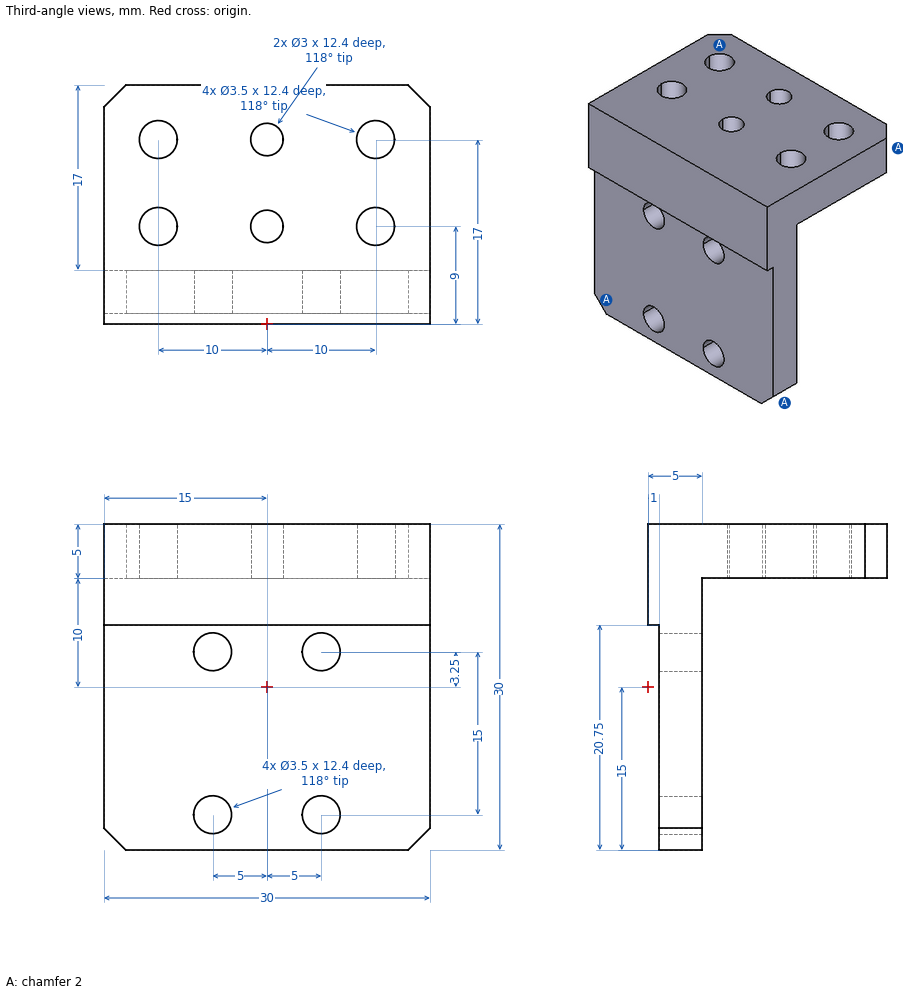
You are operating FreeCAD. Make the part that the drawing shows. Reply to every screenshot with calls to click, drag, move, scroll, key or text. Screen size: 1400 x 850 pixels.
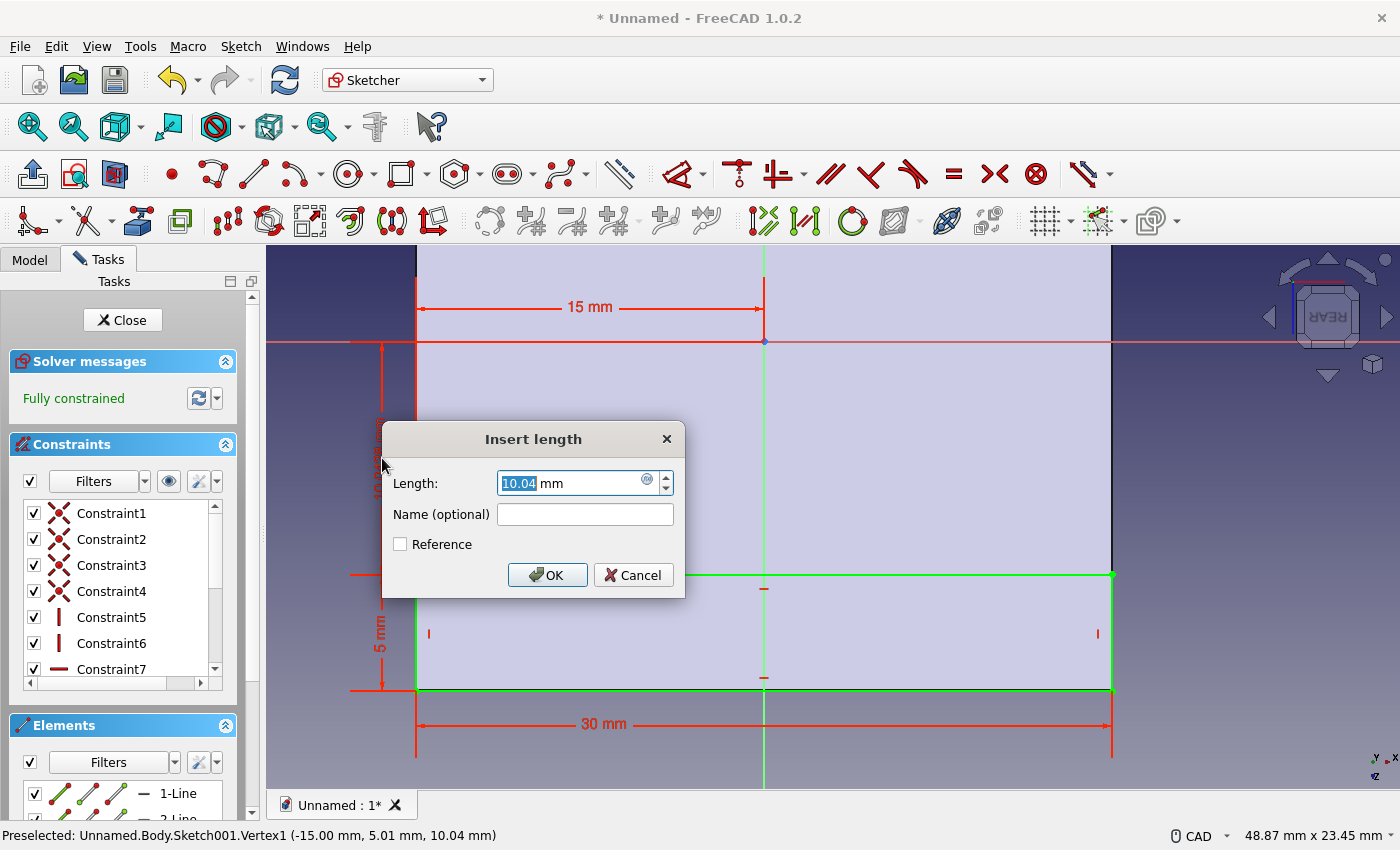
text(10)
key(Return)
key(Escape)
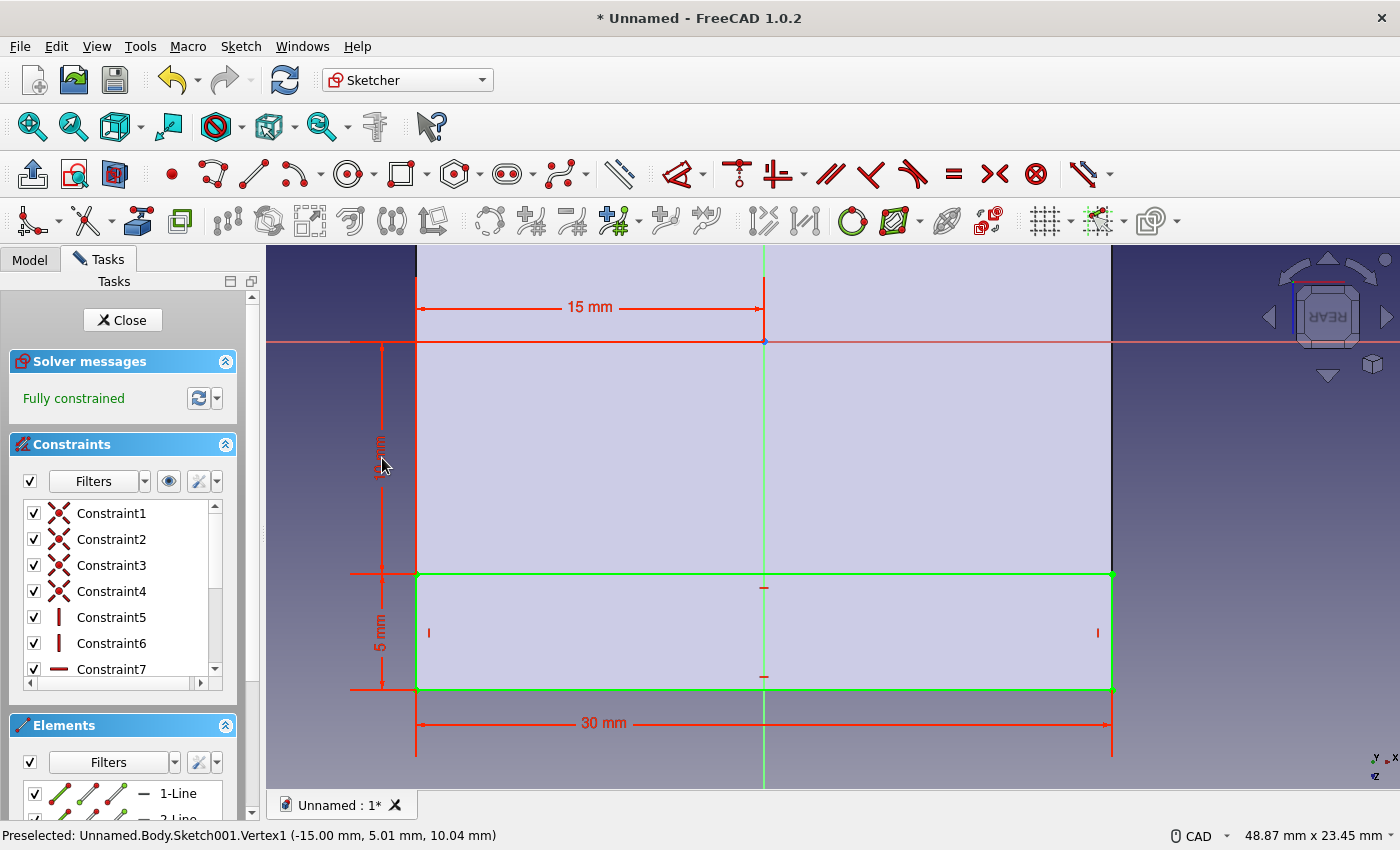
click(123, 320)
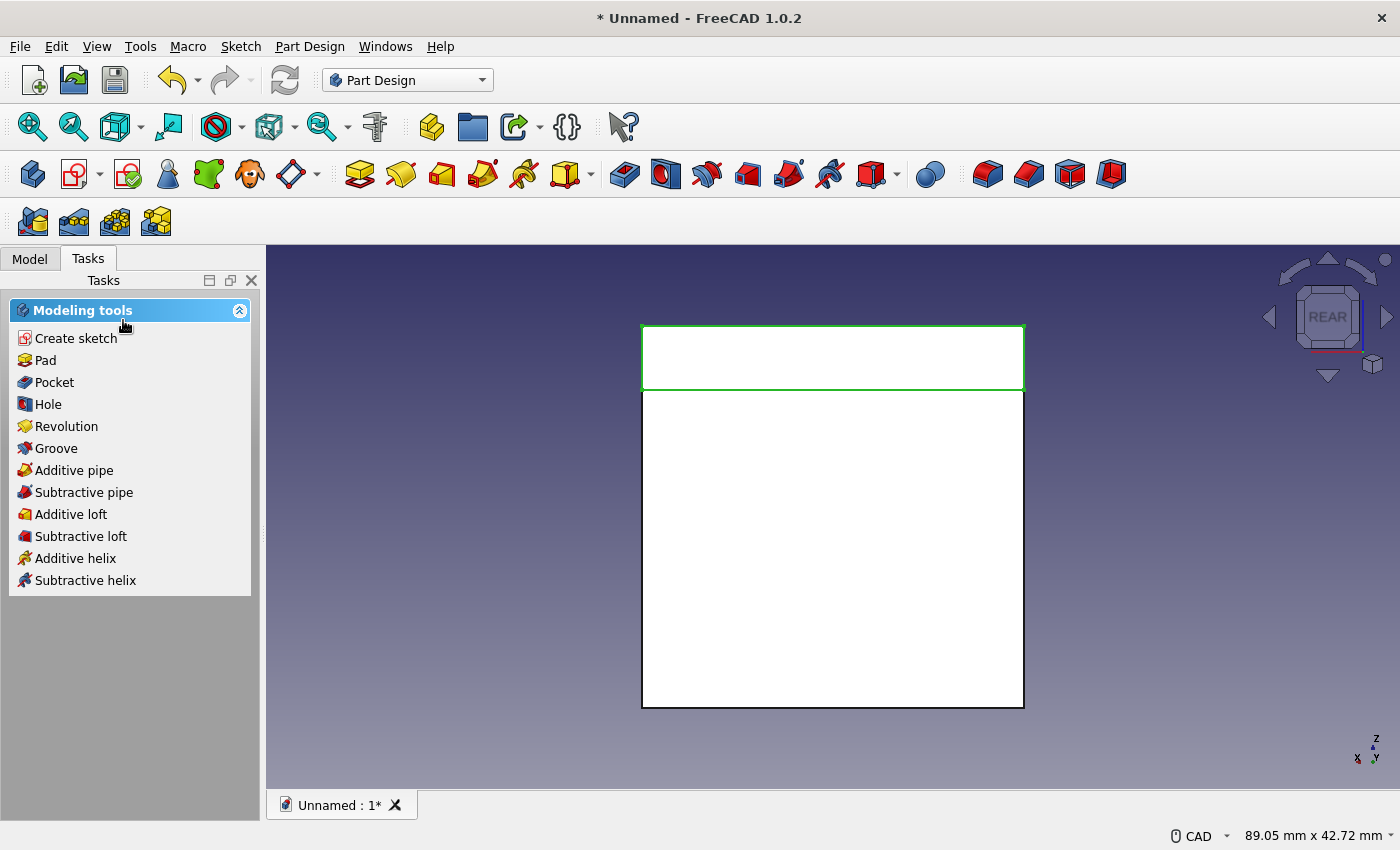
click(360, 174)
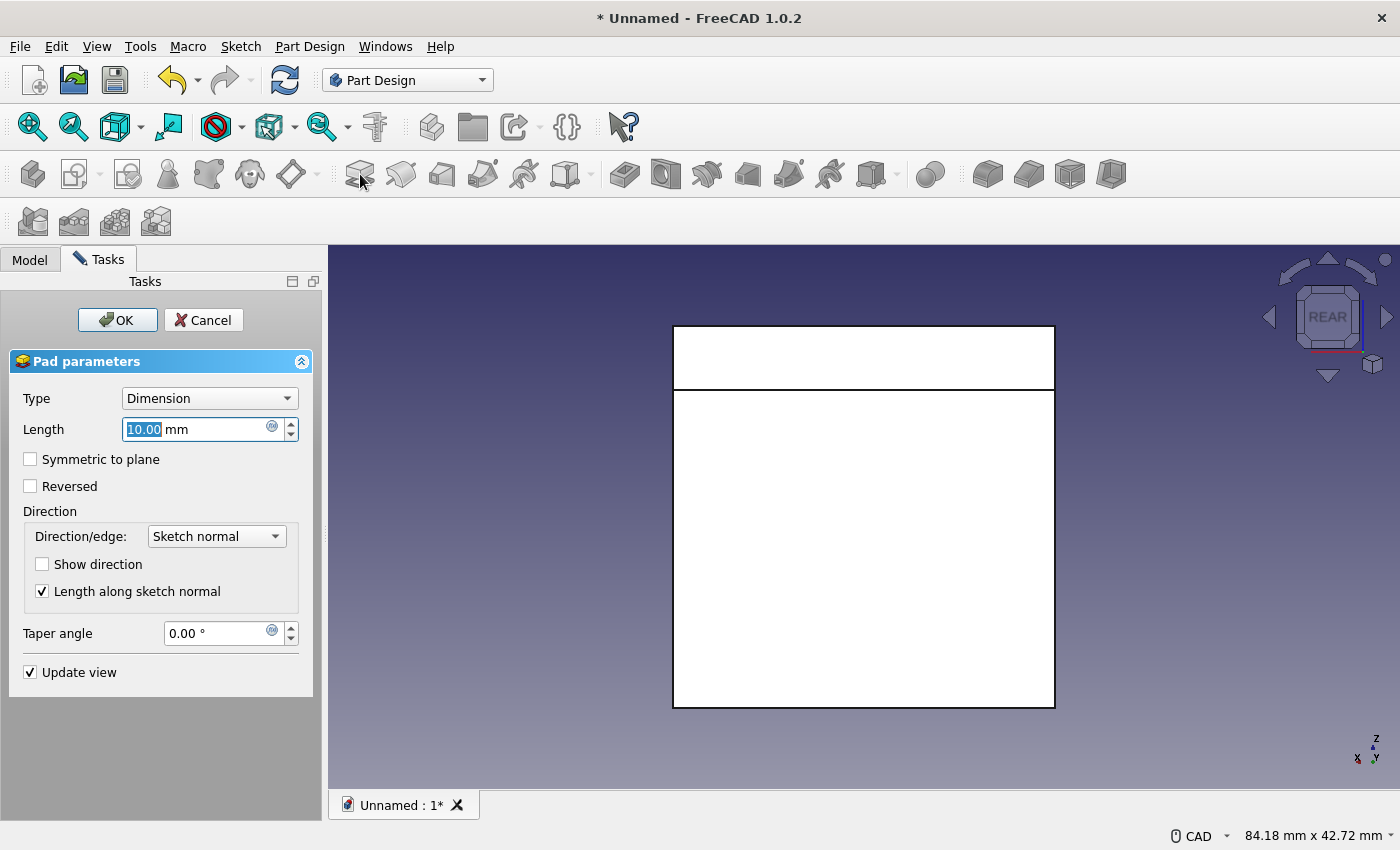
text(17)
key(Tab)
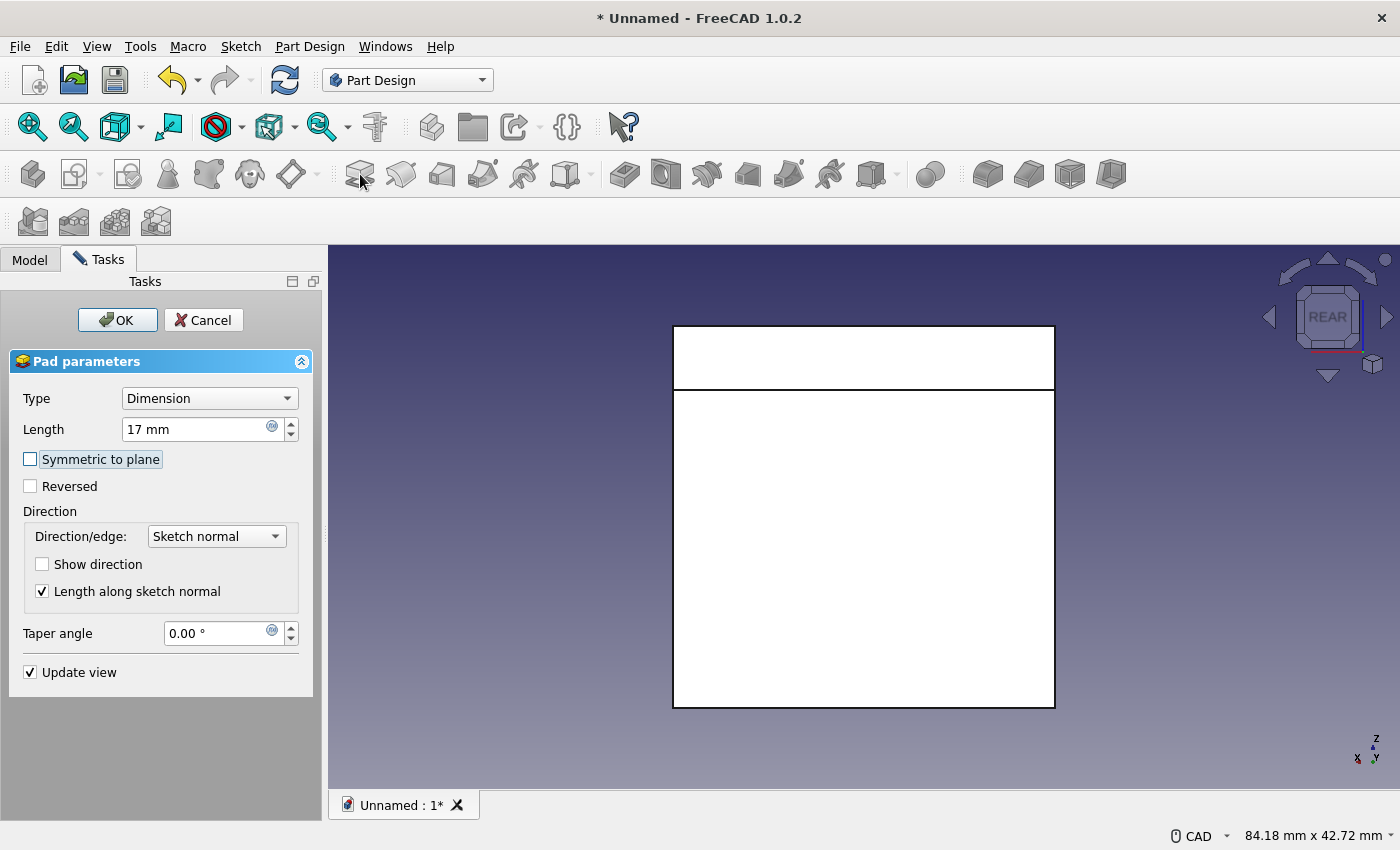
click(118, 320)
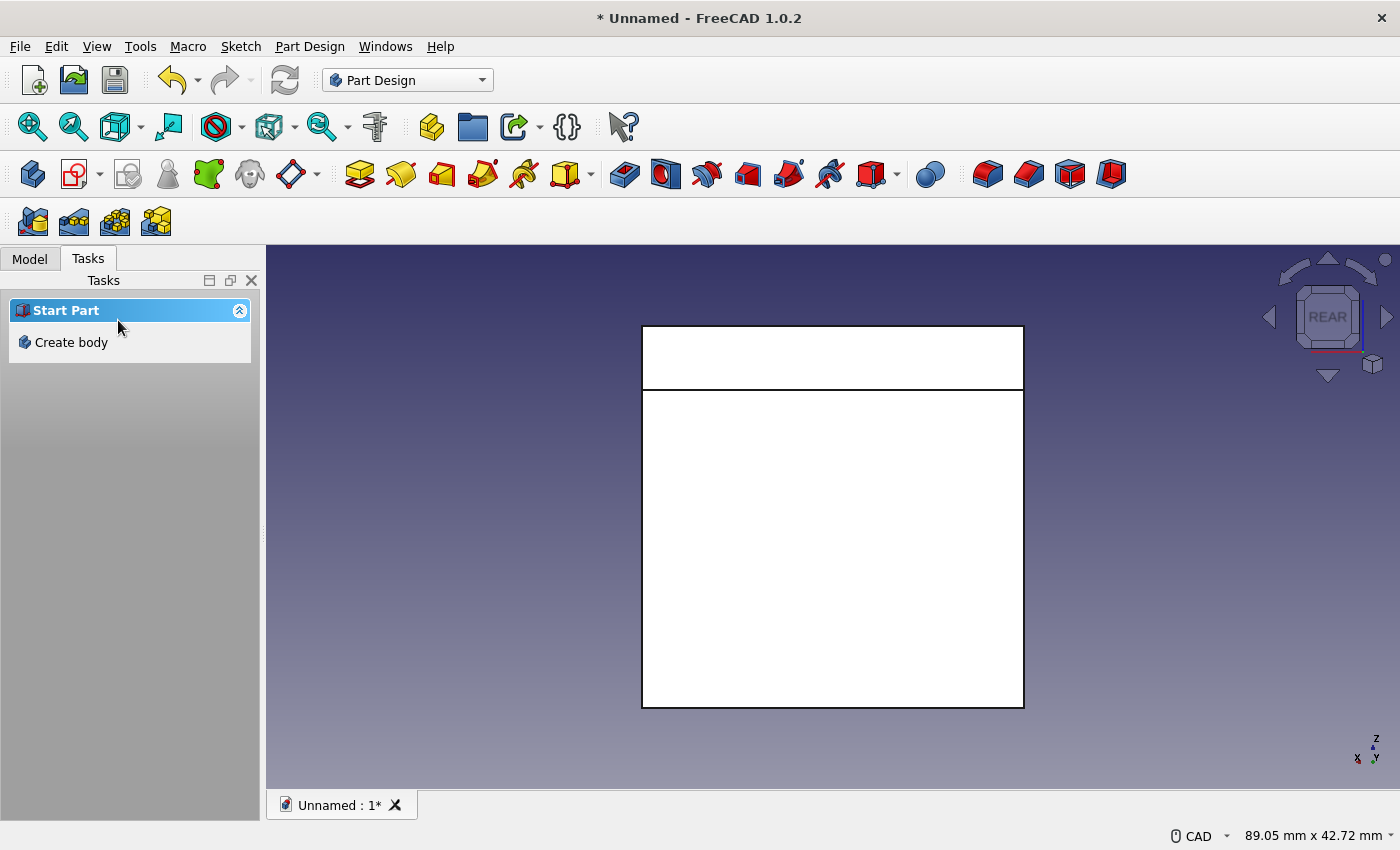
click(833, 548)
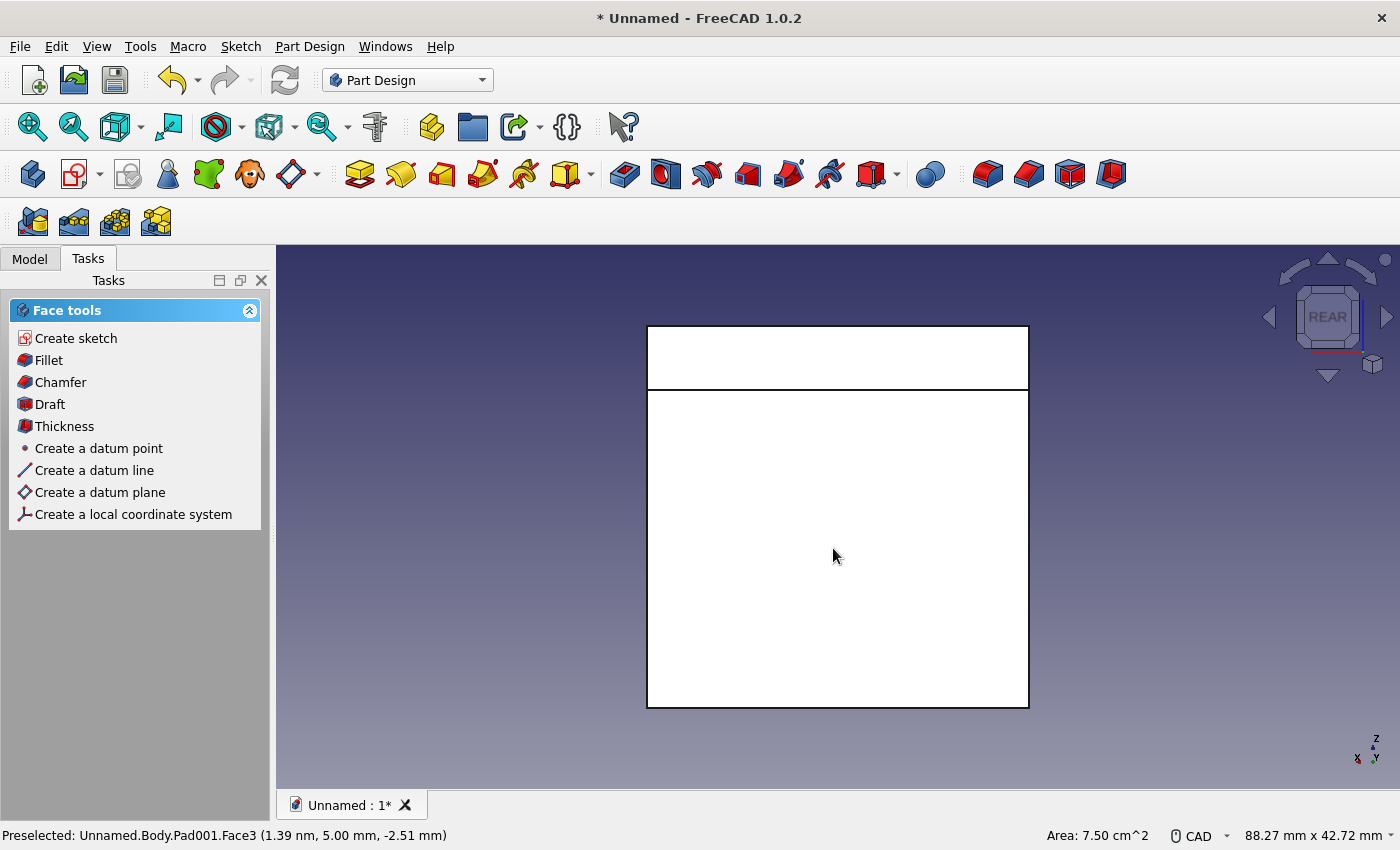
click(74, 174)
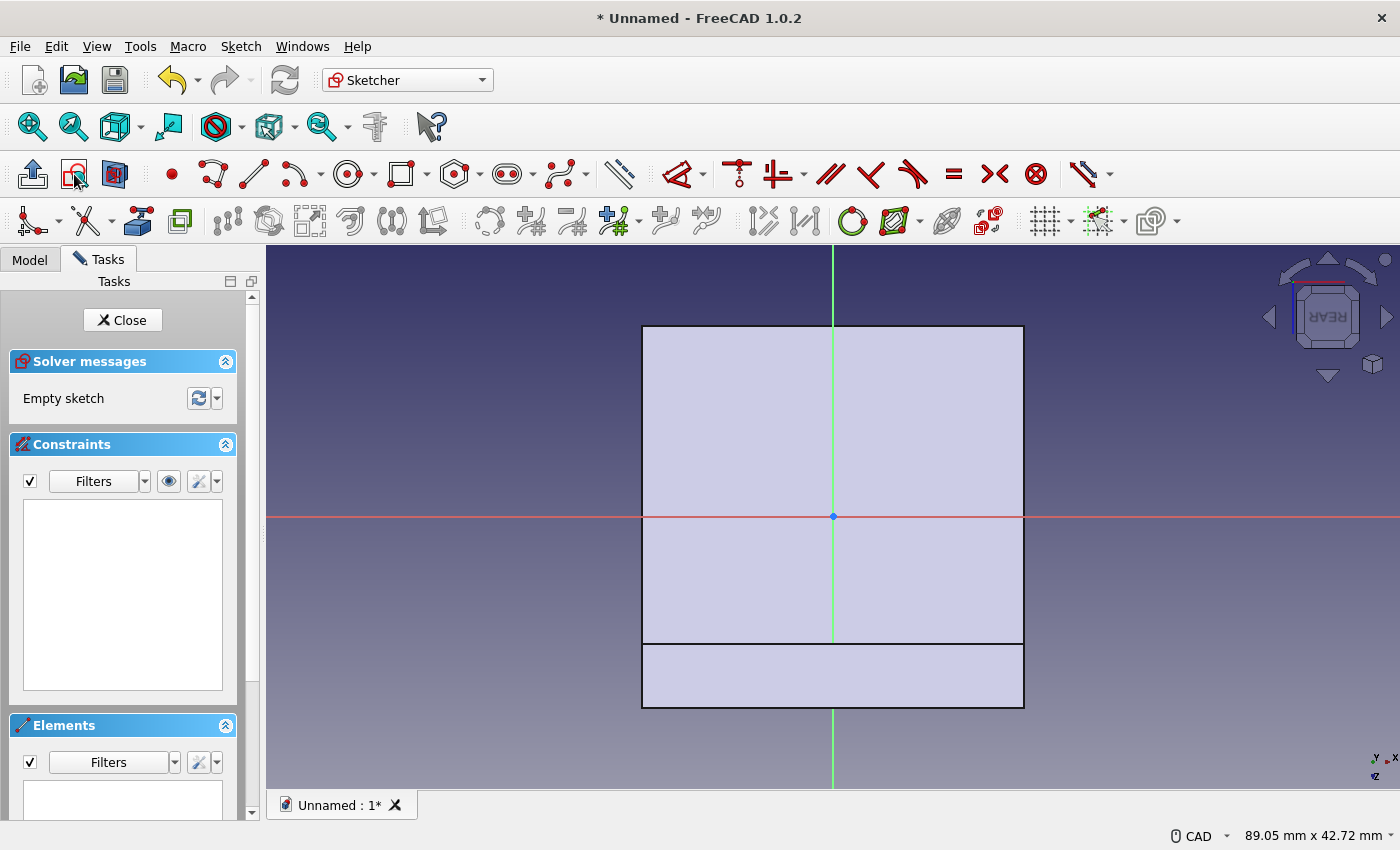
key(q)
key(s)